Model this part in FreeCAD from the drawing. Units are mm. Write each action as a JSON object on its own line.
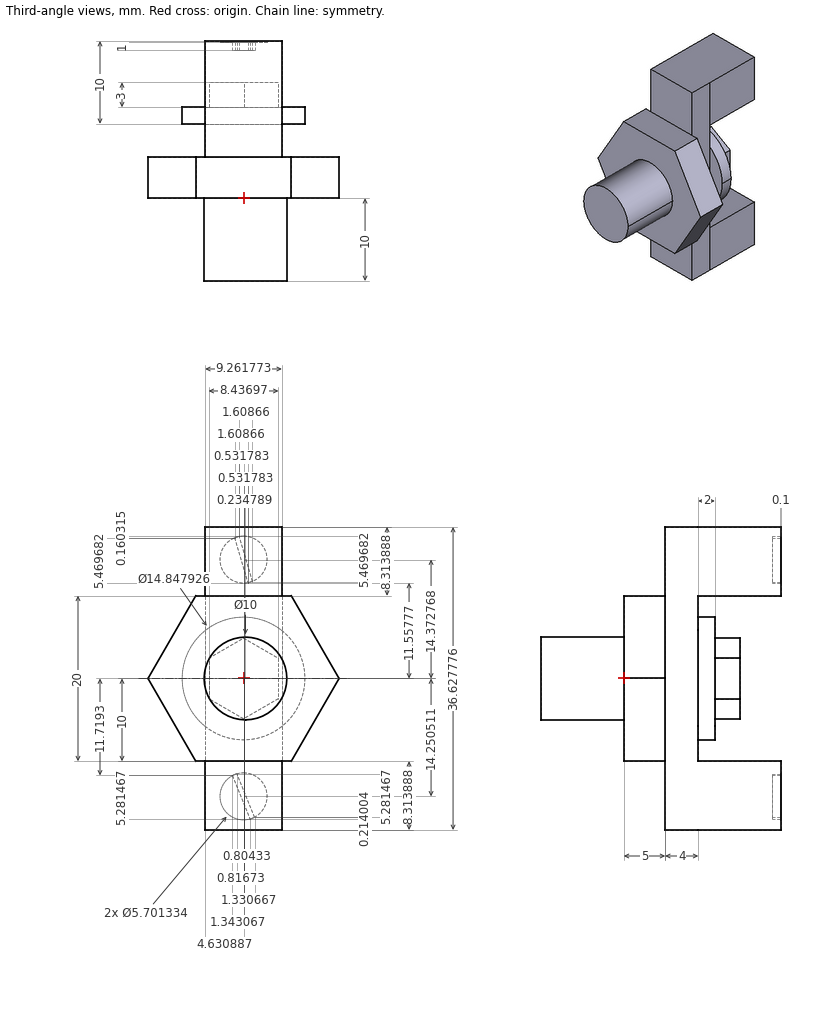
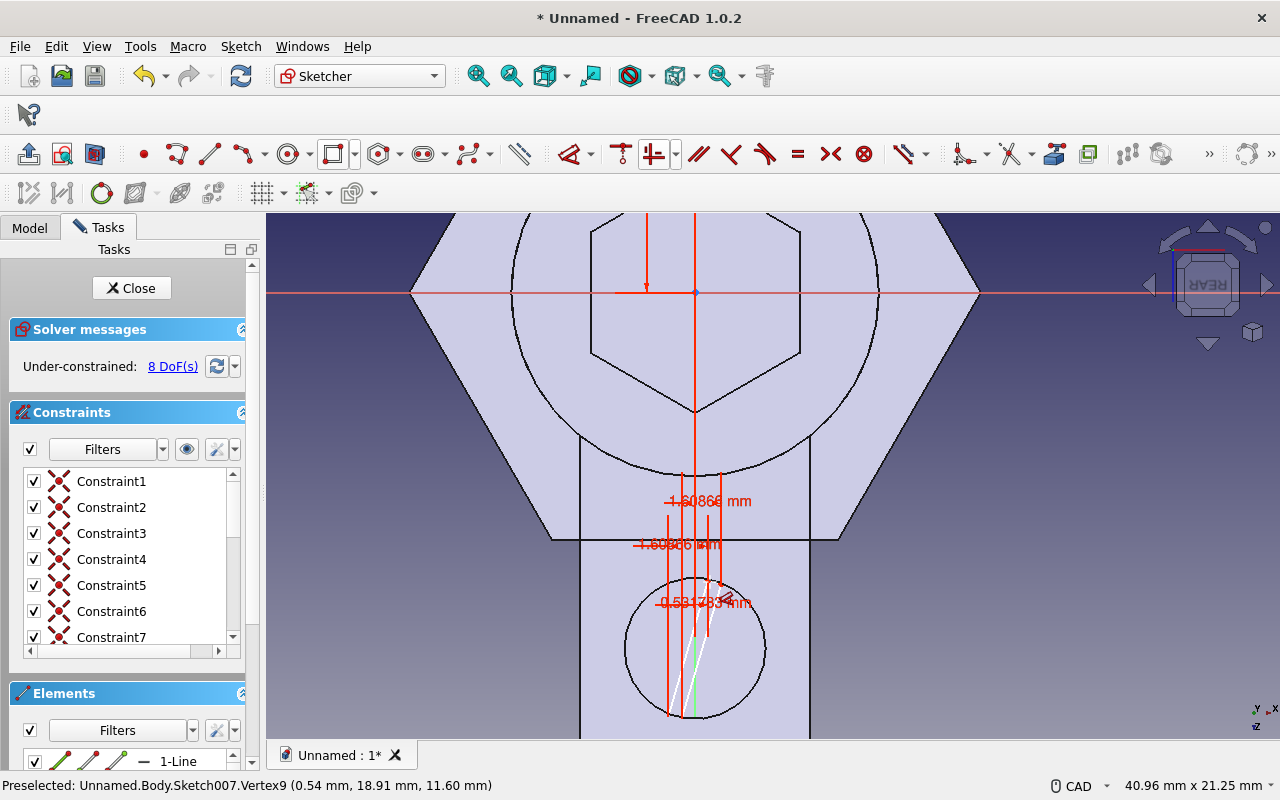
{"action": "left_click", "coordinate": [708, 580]}
{"action": "left_click", "coordinate": [742, 436]}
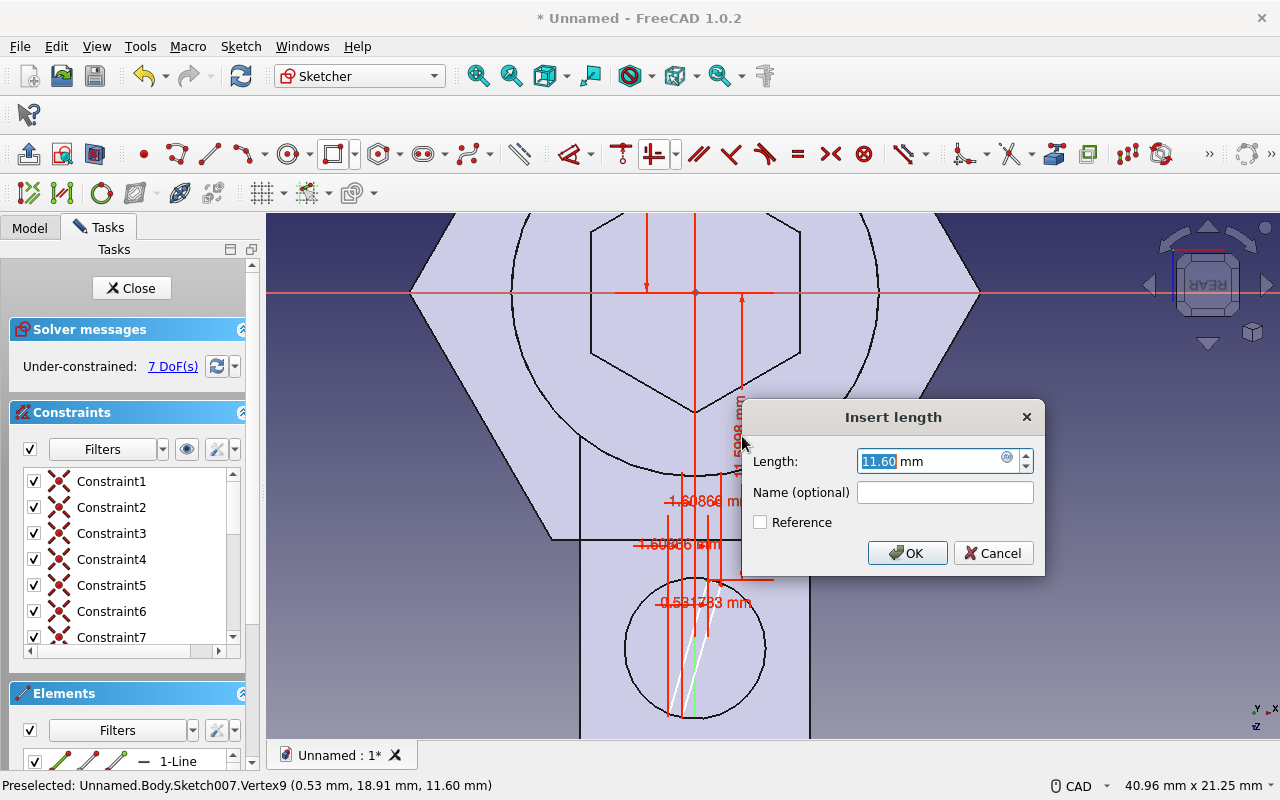
{"action": "type", "text": "11.55777"}
{"action": "key", "text": "Return"}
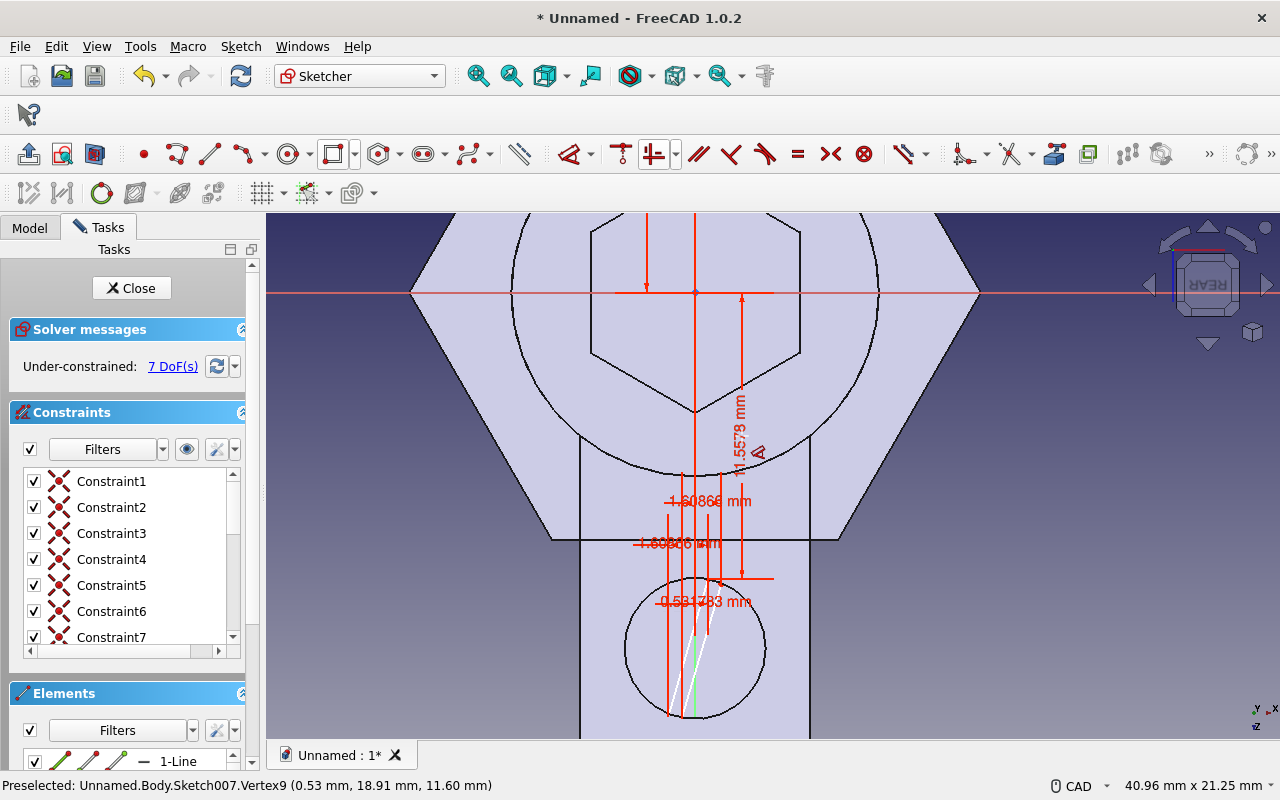
{"action": "scroll", "coordinate": [710, 581], "scroll_direction": "down", "scroll_amount": 5}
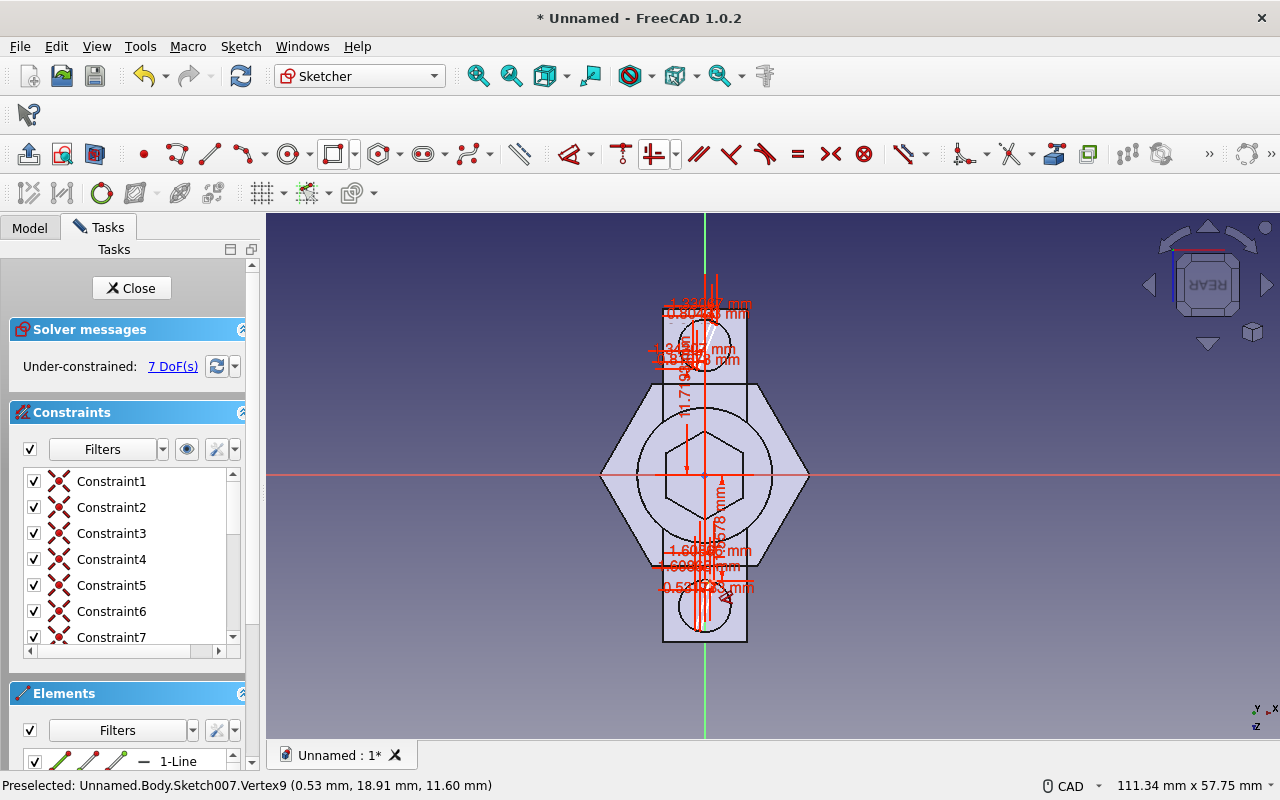
{"action": "scroll", "coordinate": [700, 632], "scroll_direction": "up", "scroll_amount": 11}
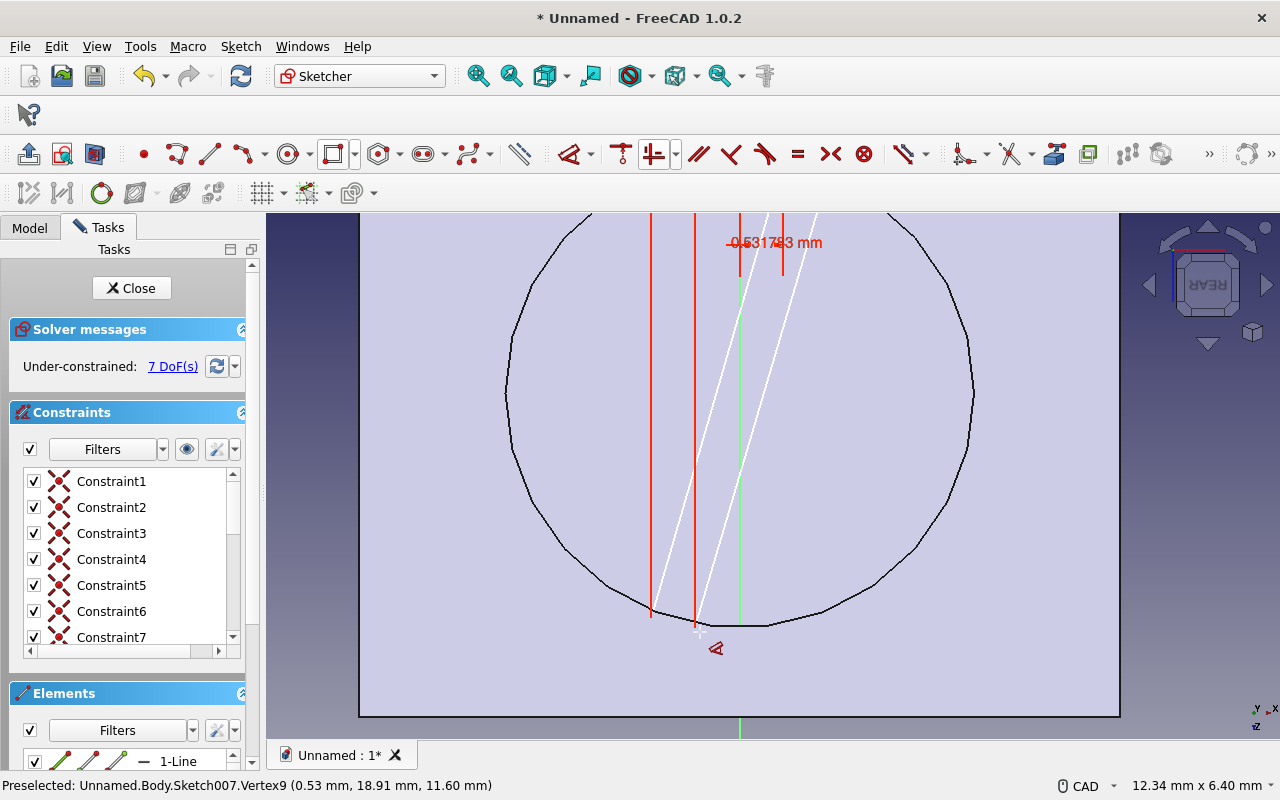
{"action": "left_click", "coordinate": [695, 628]}
{"action": "left_click", "coordinate": [717, 662]}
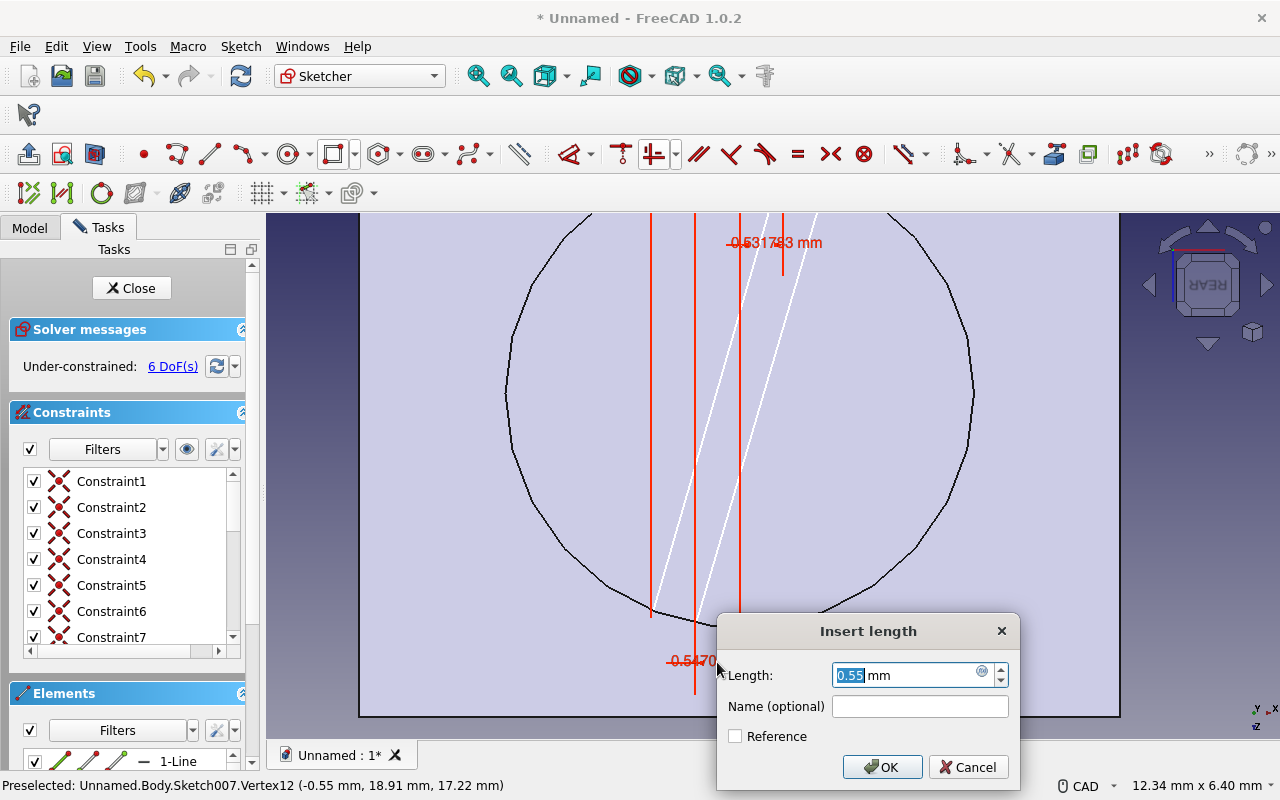
{"action": "type", "text": "0.531783"}
{"action": "key", "text": "Return"}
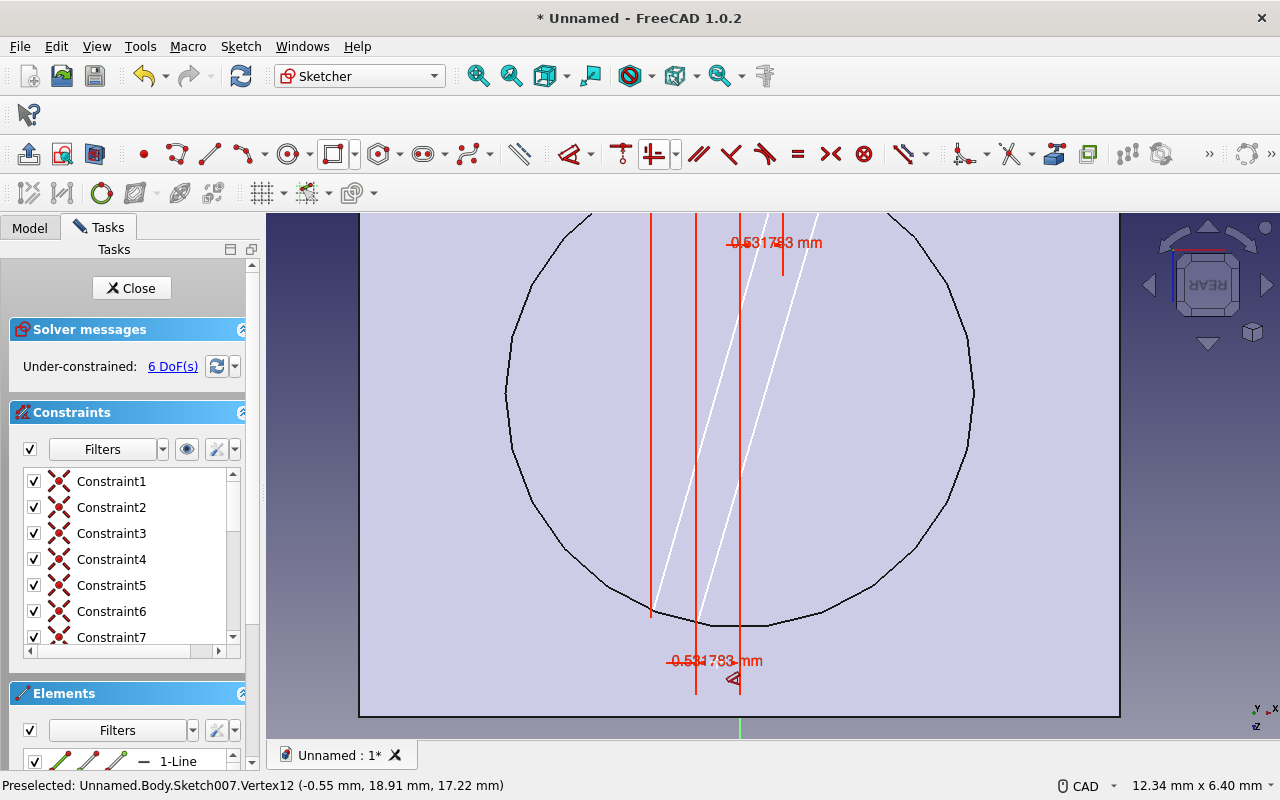
{"action": "scroll", "coordinate": [700, 633], "scroll_direction": "down", "scroll_amount": 11}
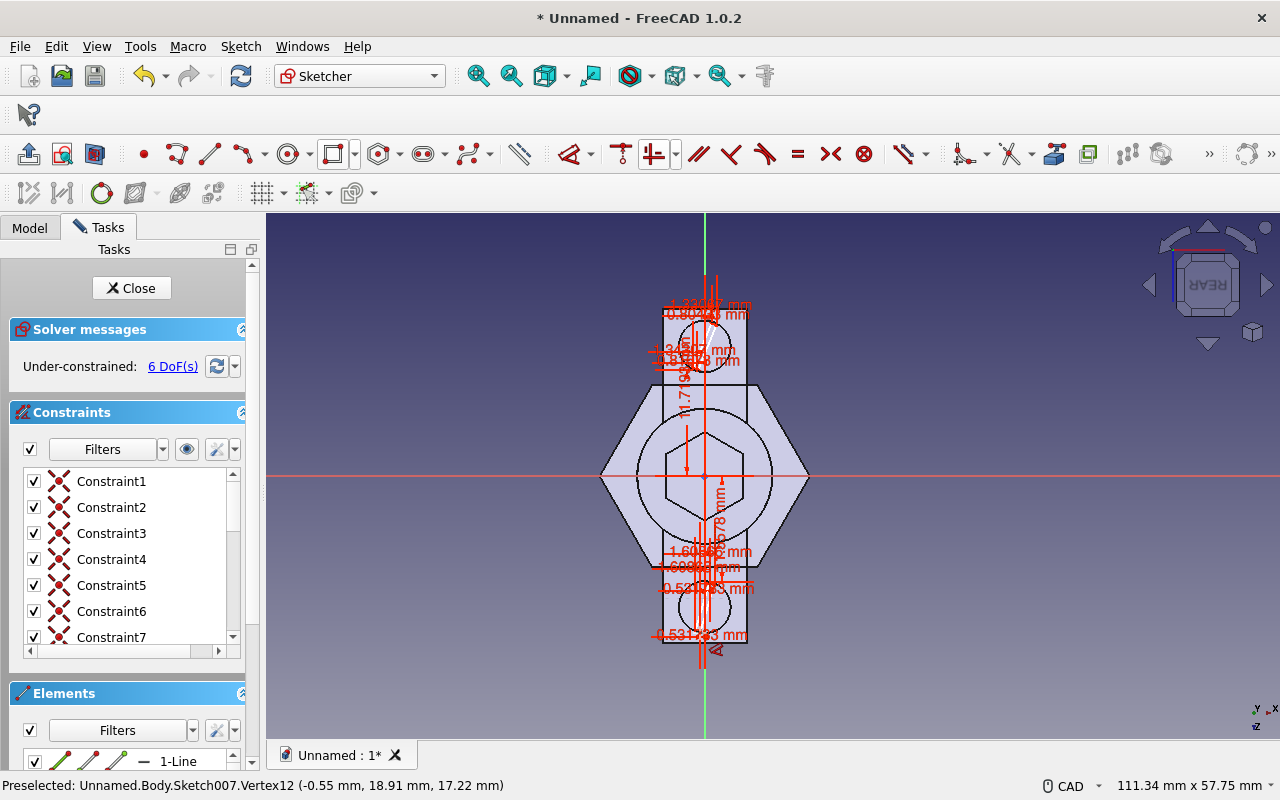
{"action": "scroll", "coordinate": [703, 358], "scroll_direction": "up", "scroll_amount": 11}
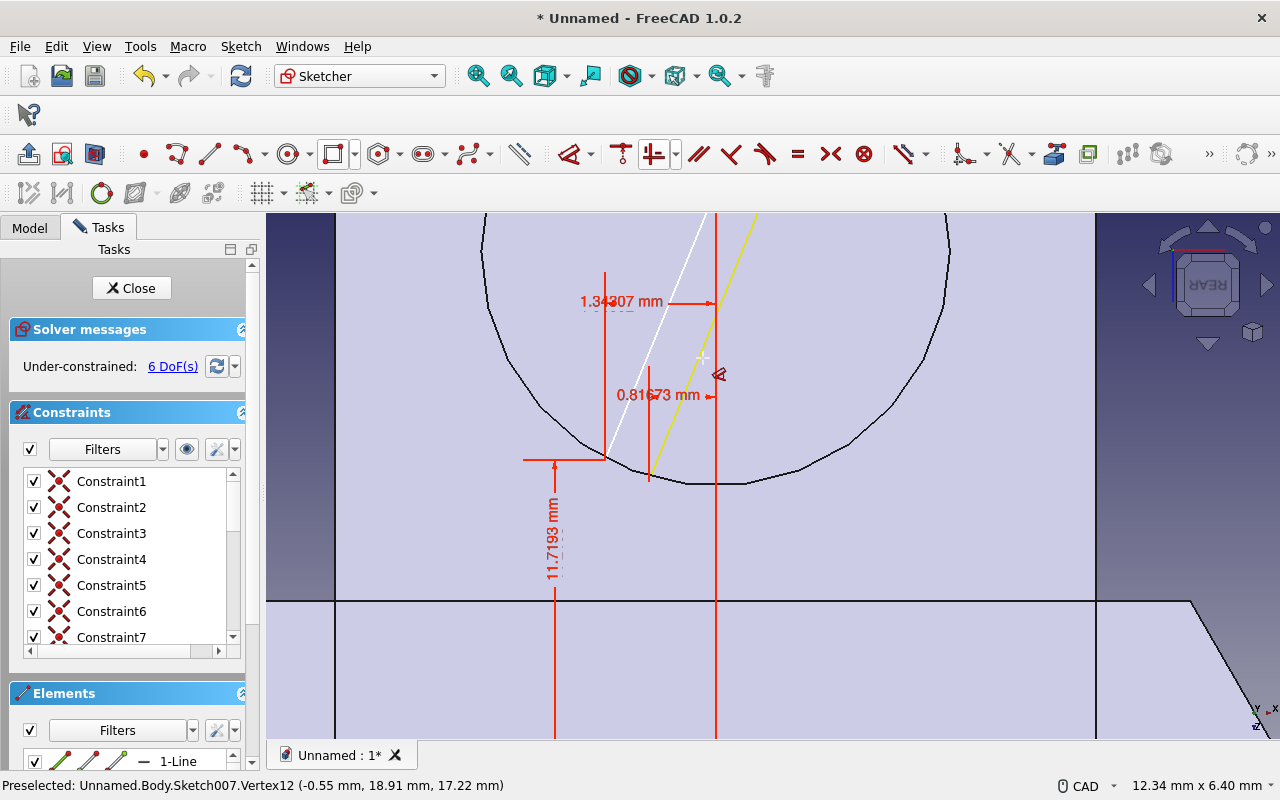
{"action": "left_click", "coordinate": [701, 352]}
{"action": "left_click", "coordinate": [859, 362]}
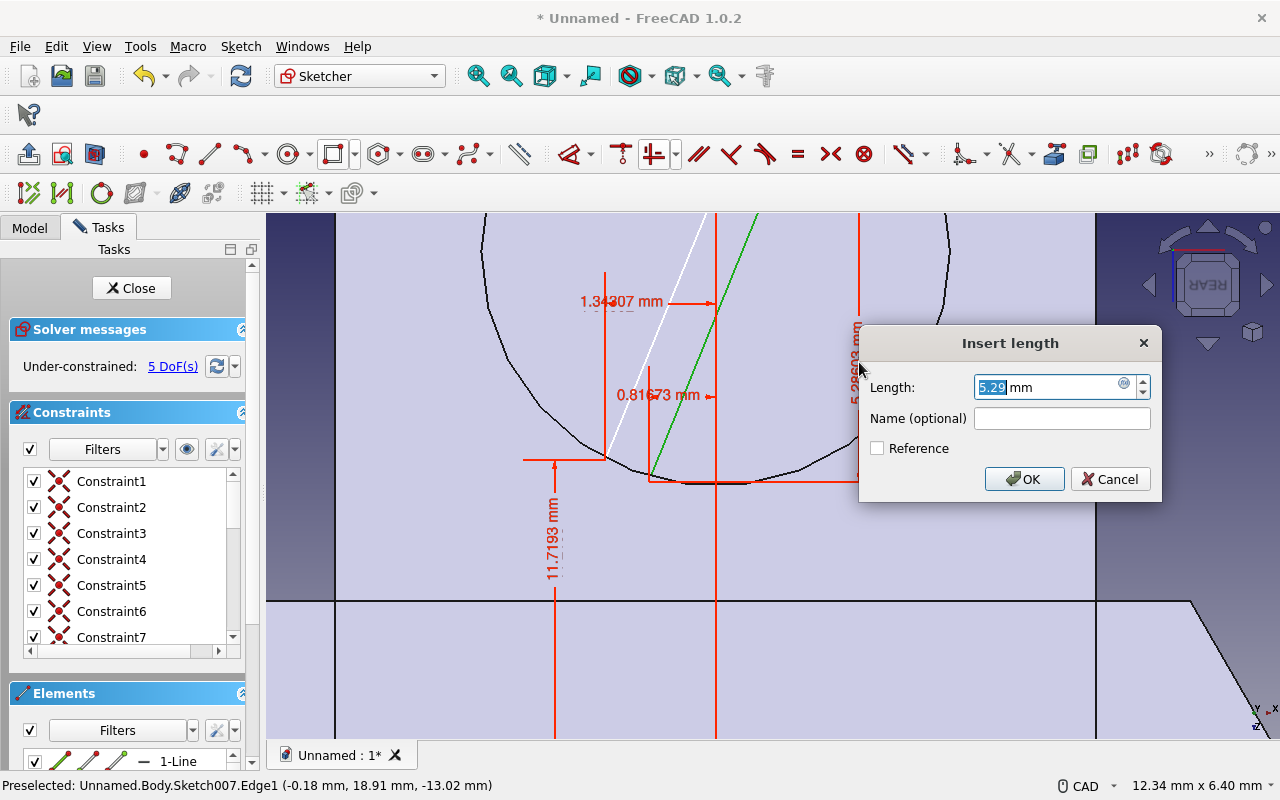
{"action": "type", "text": "5.281467"}
{"action": "key", "text": "Return"}